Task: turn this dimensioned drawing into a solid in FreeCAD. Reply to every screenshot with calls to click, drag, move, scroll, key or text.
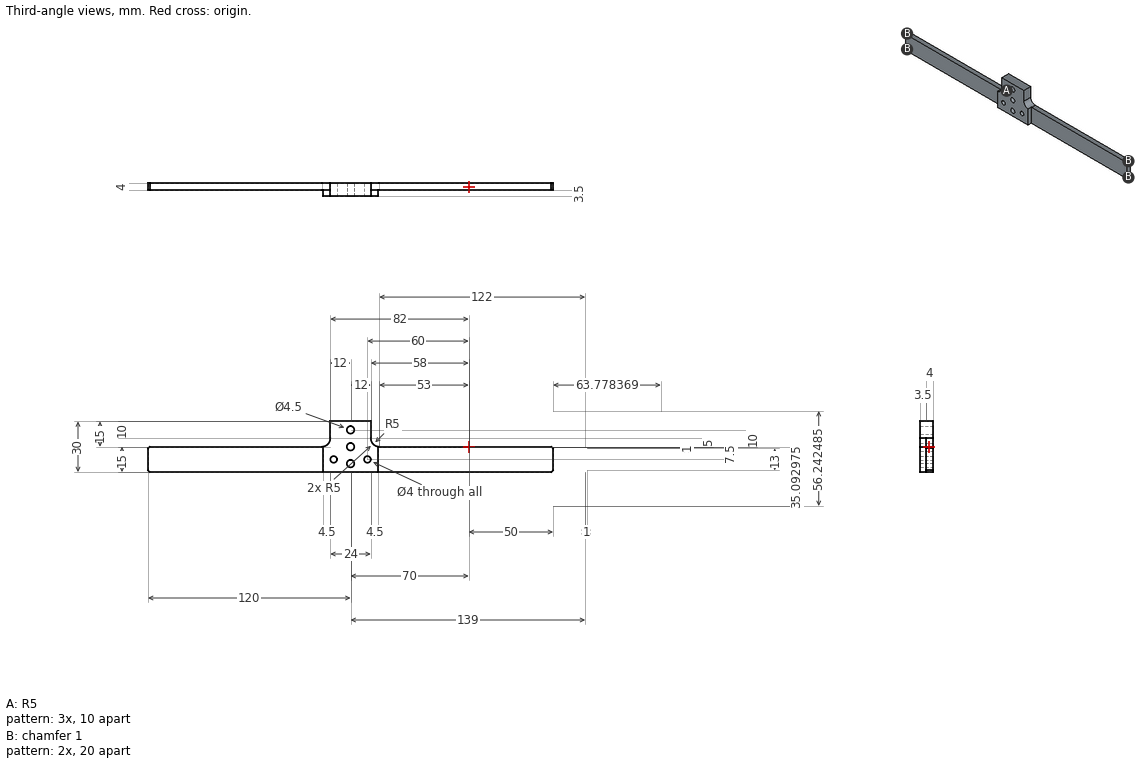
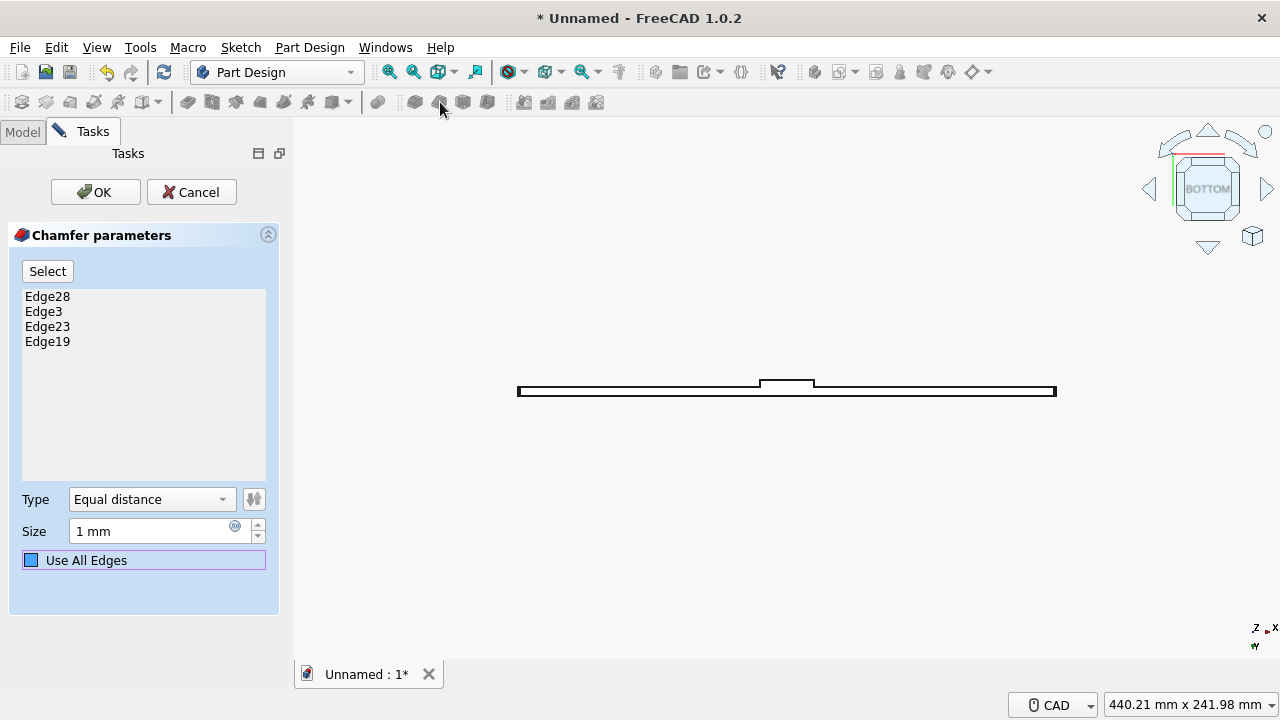
click(96, 192)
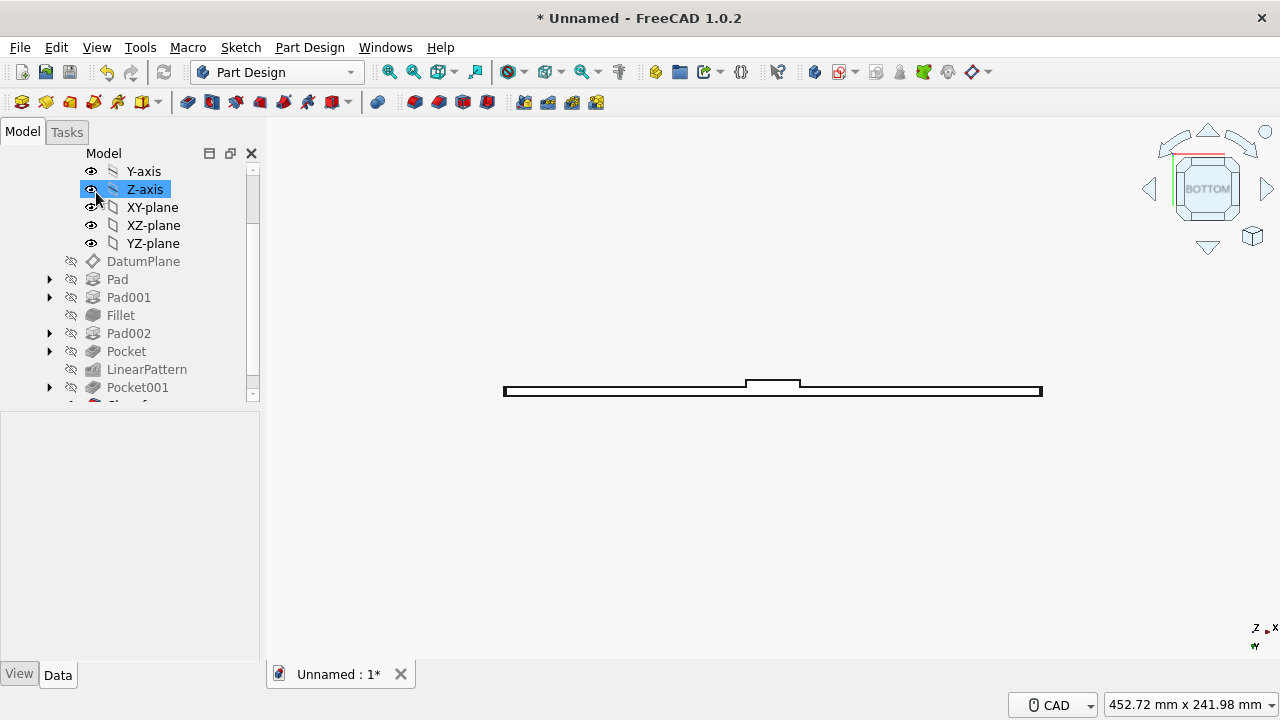
key(0)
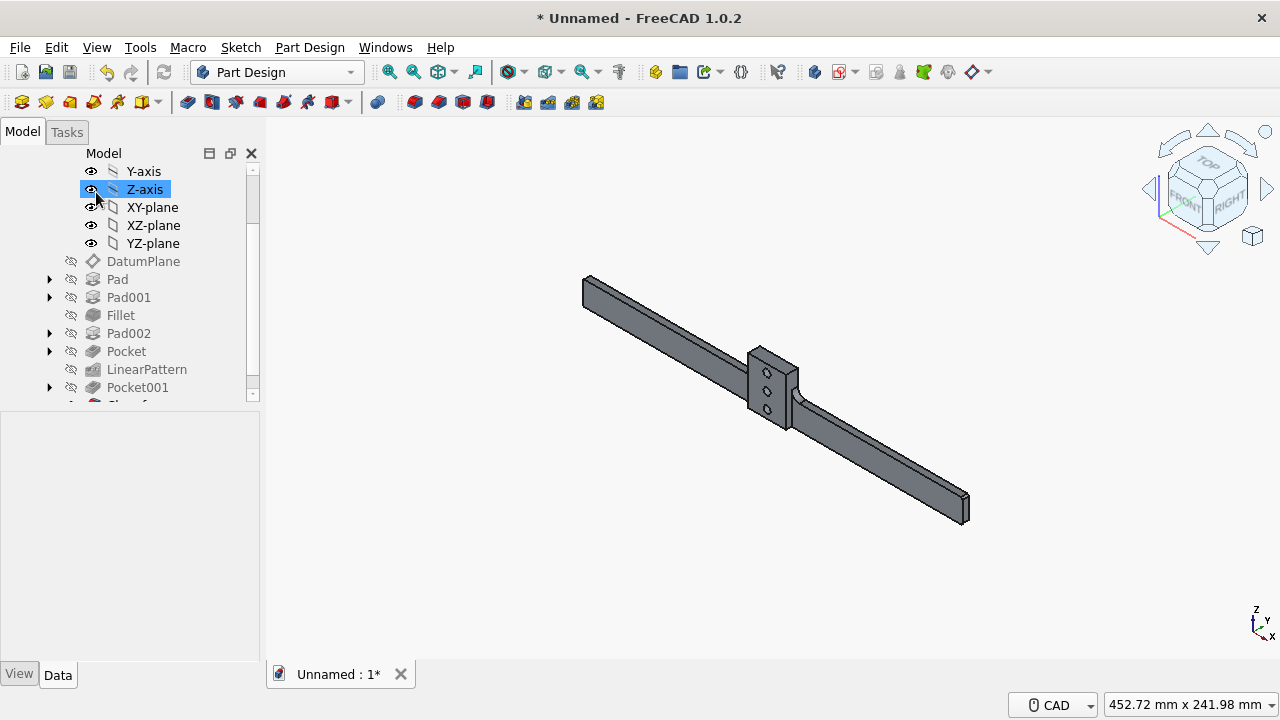
click(778, 389)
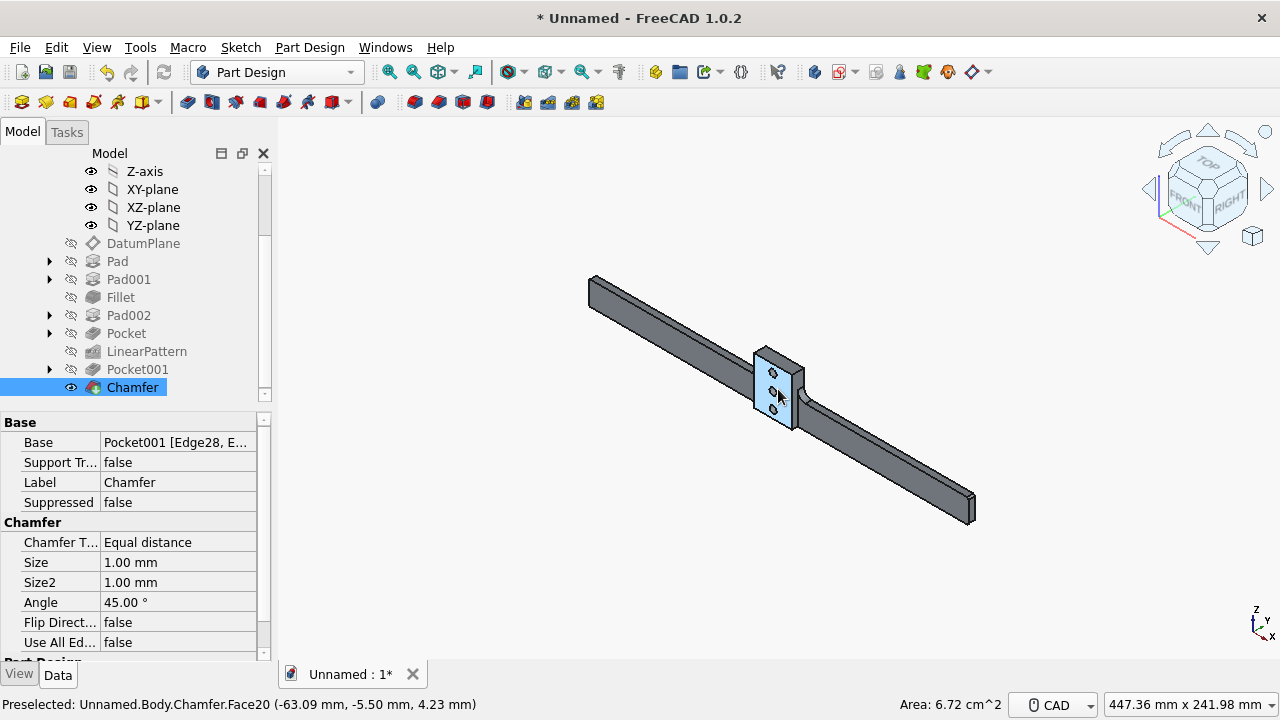
click(840, 72)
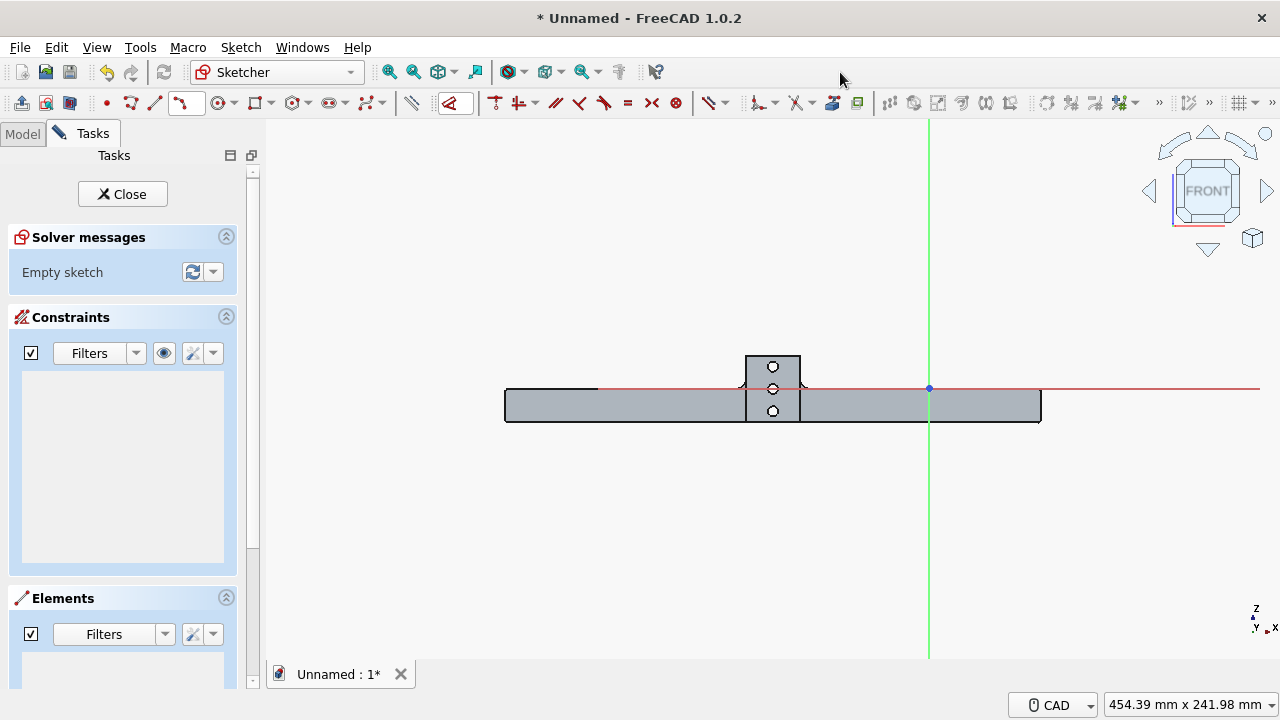
scroll(790, 389, up, 8)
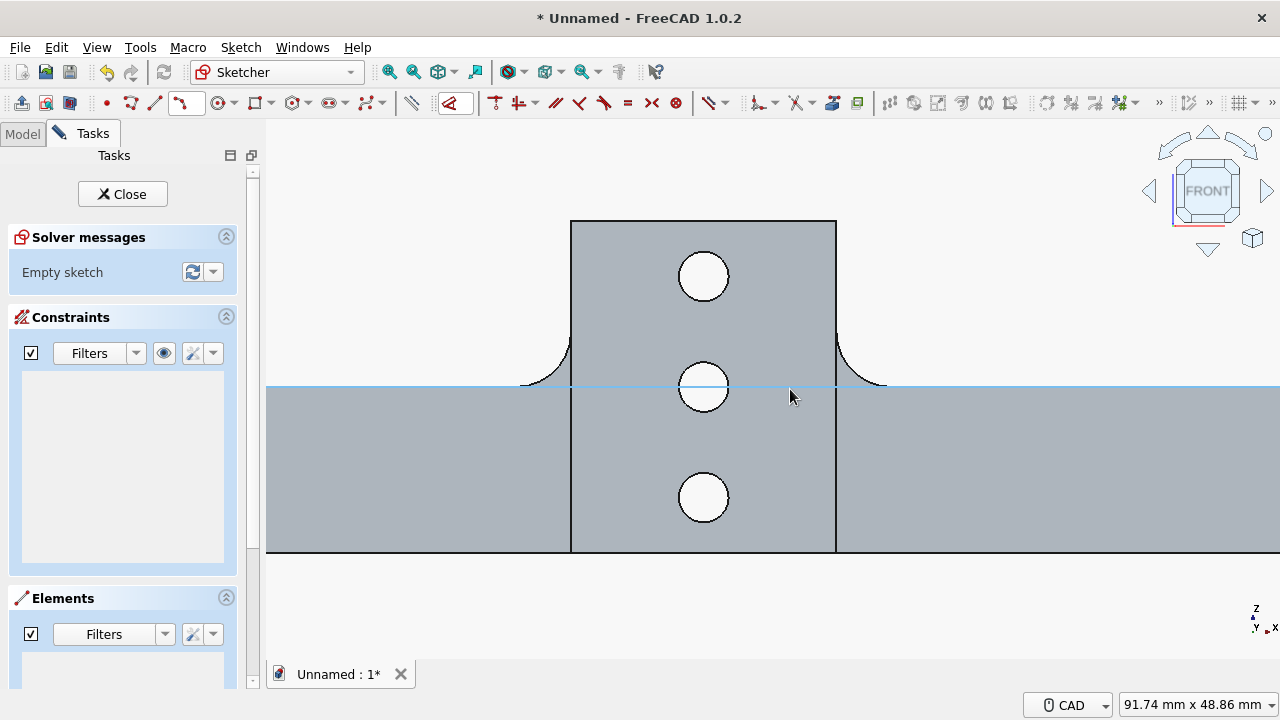
click(256, 104)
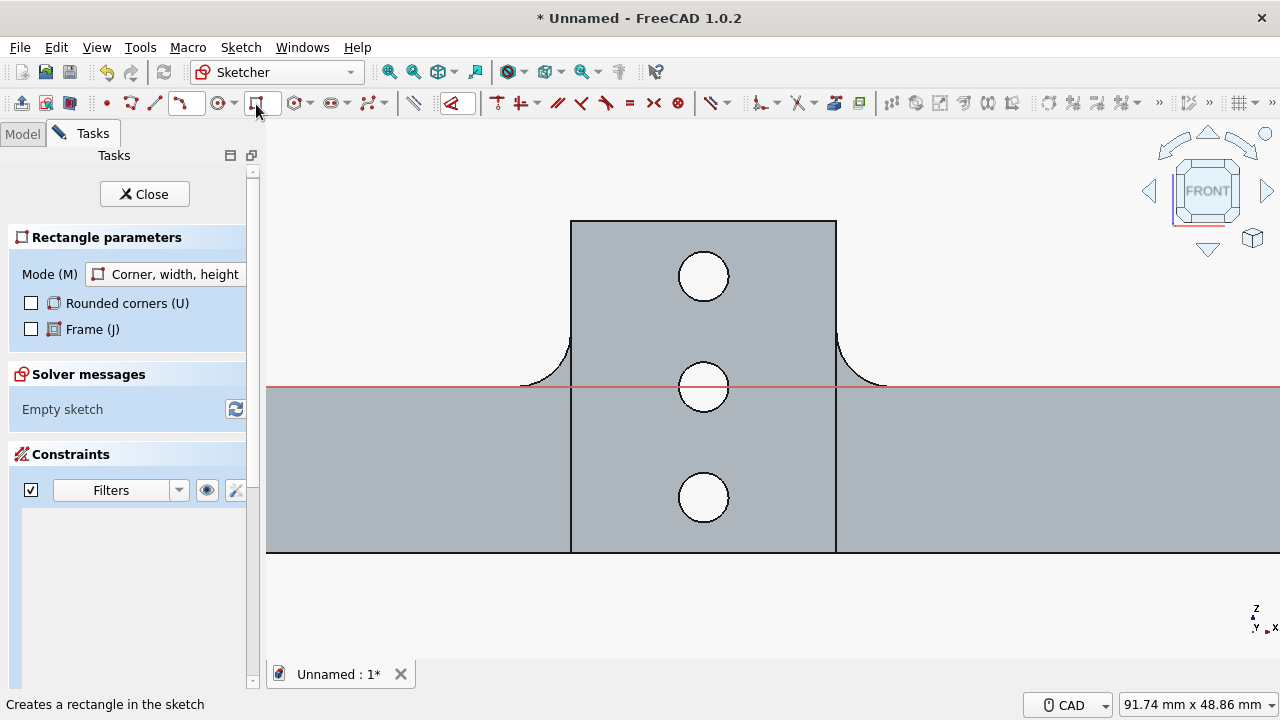
click(836, 221)
click(886, 553)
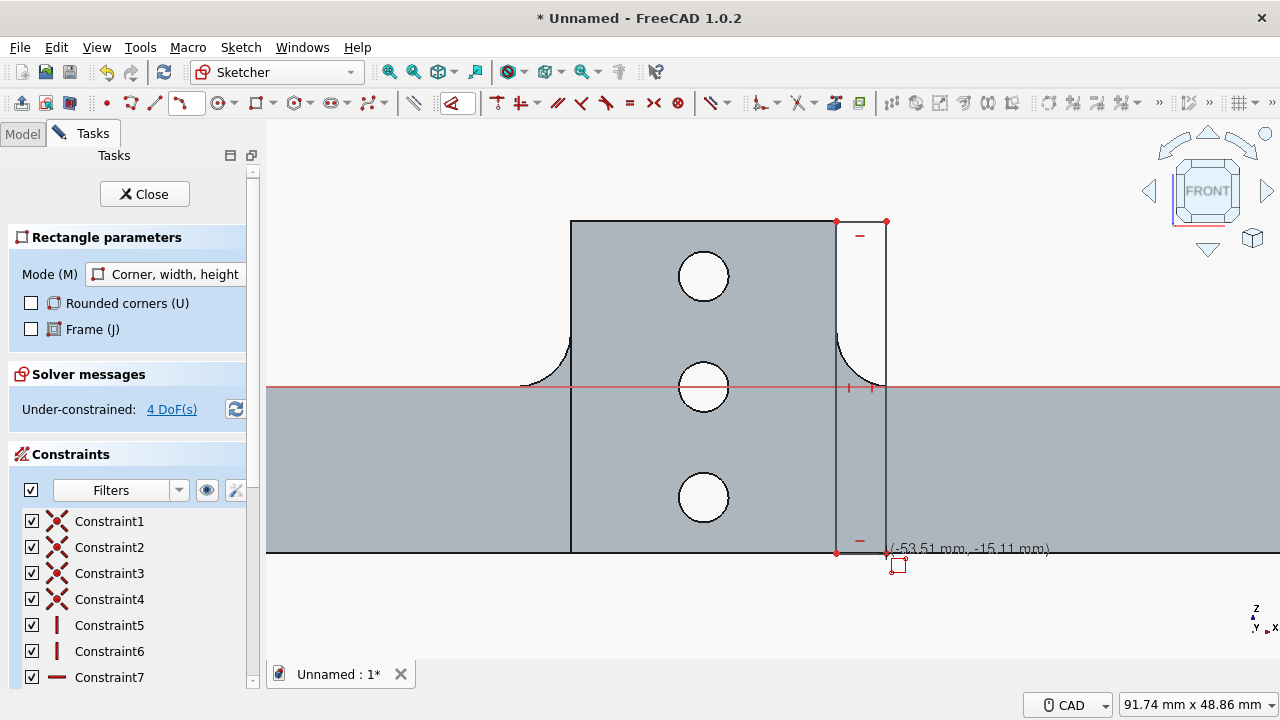
click(521, 221)
click(571, 553)
key(Escape)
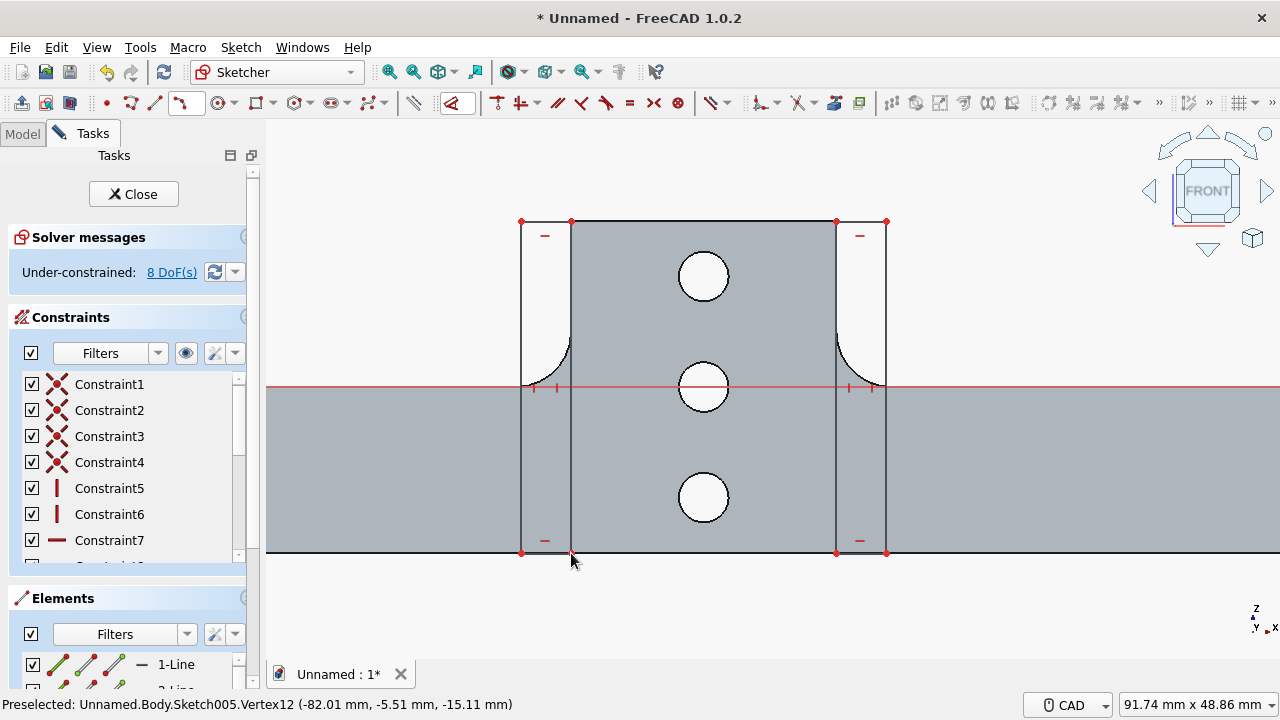
click(836, 322)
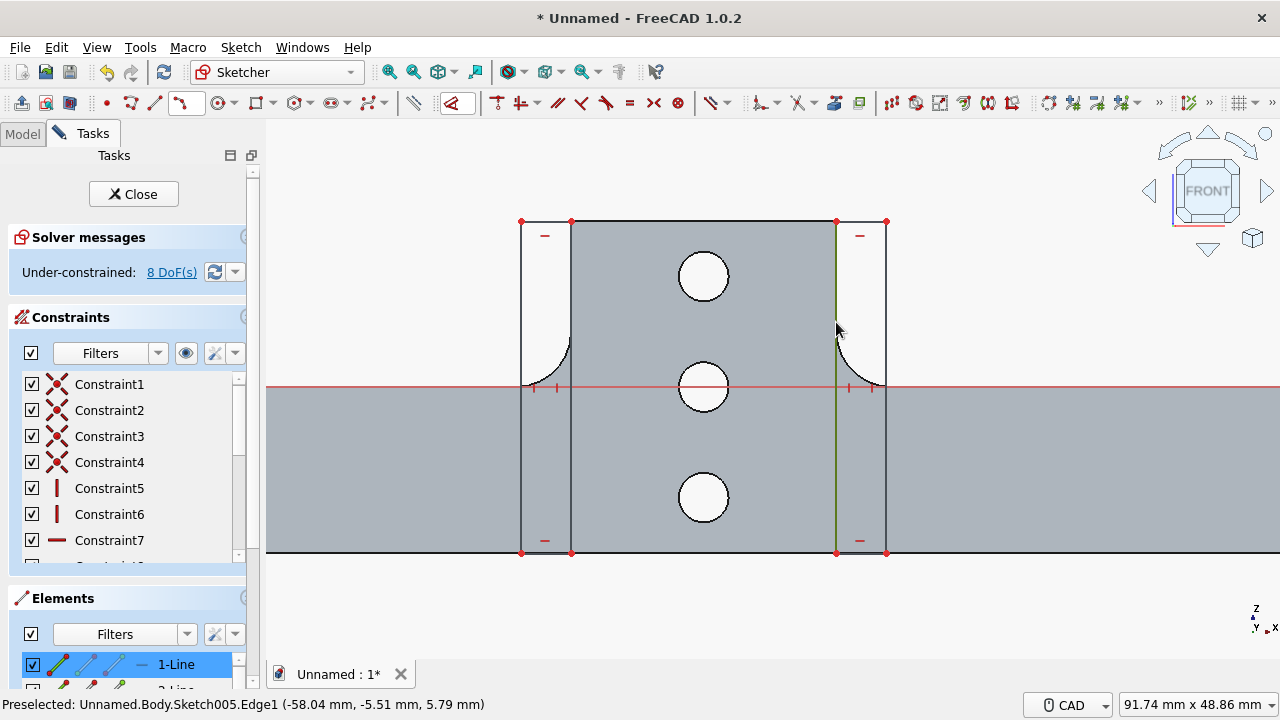
key(i)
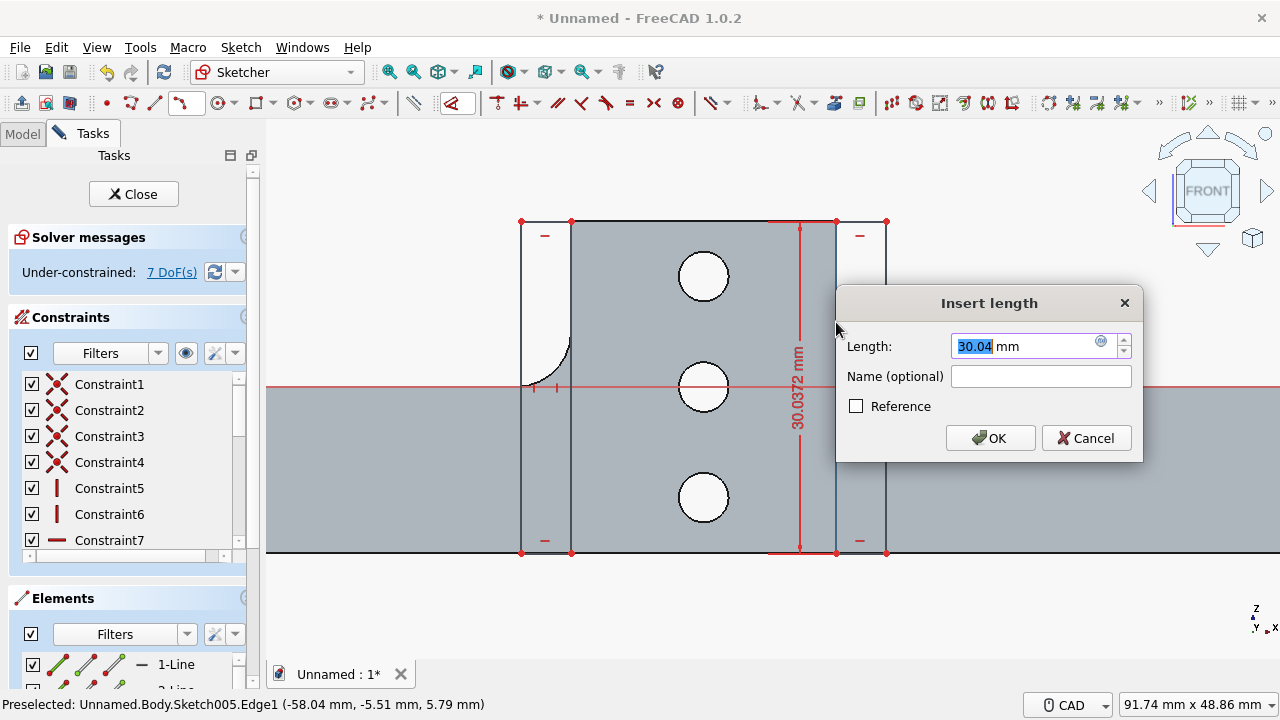
text(30)
key(Return)